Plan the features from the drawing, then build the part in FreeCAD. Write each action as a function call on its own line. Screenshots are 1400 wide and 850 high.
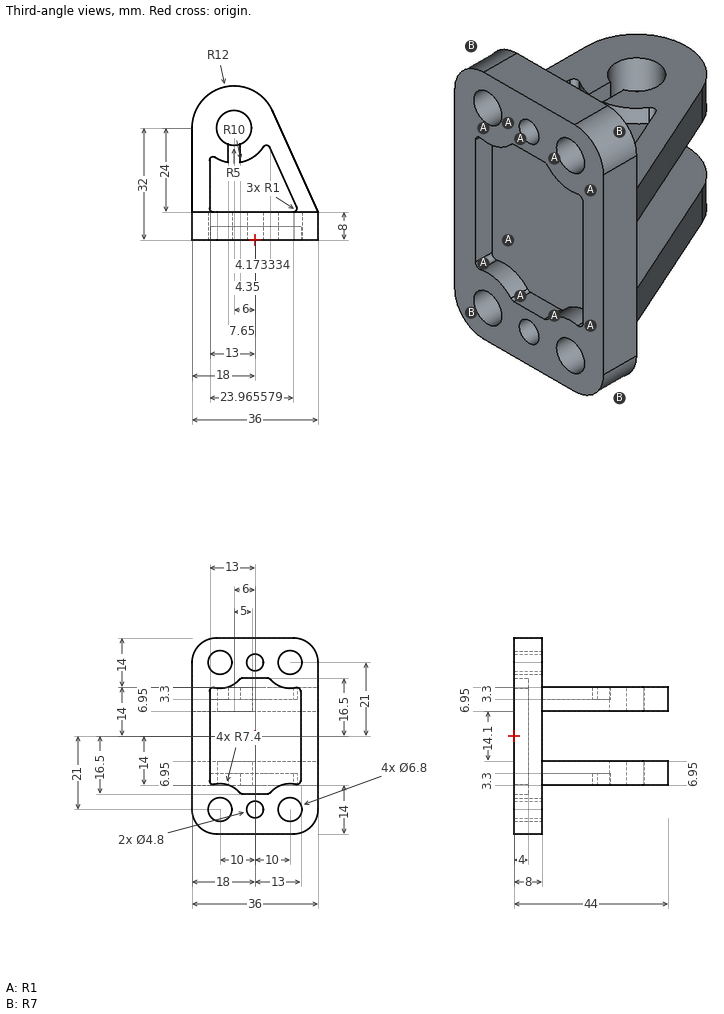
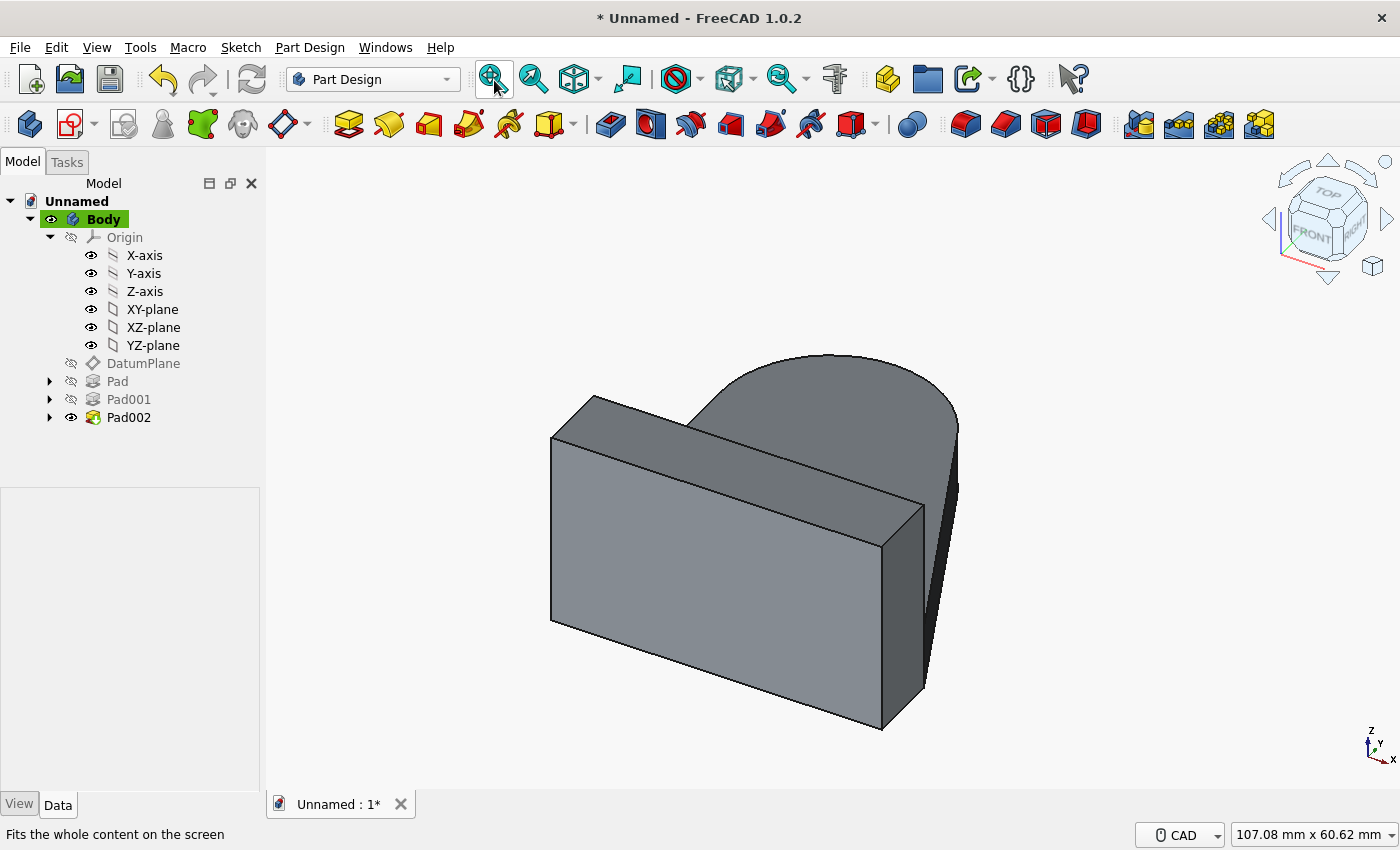
click(832, 502)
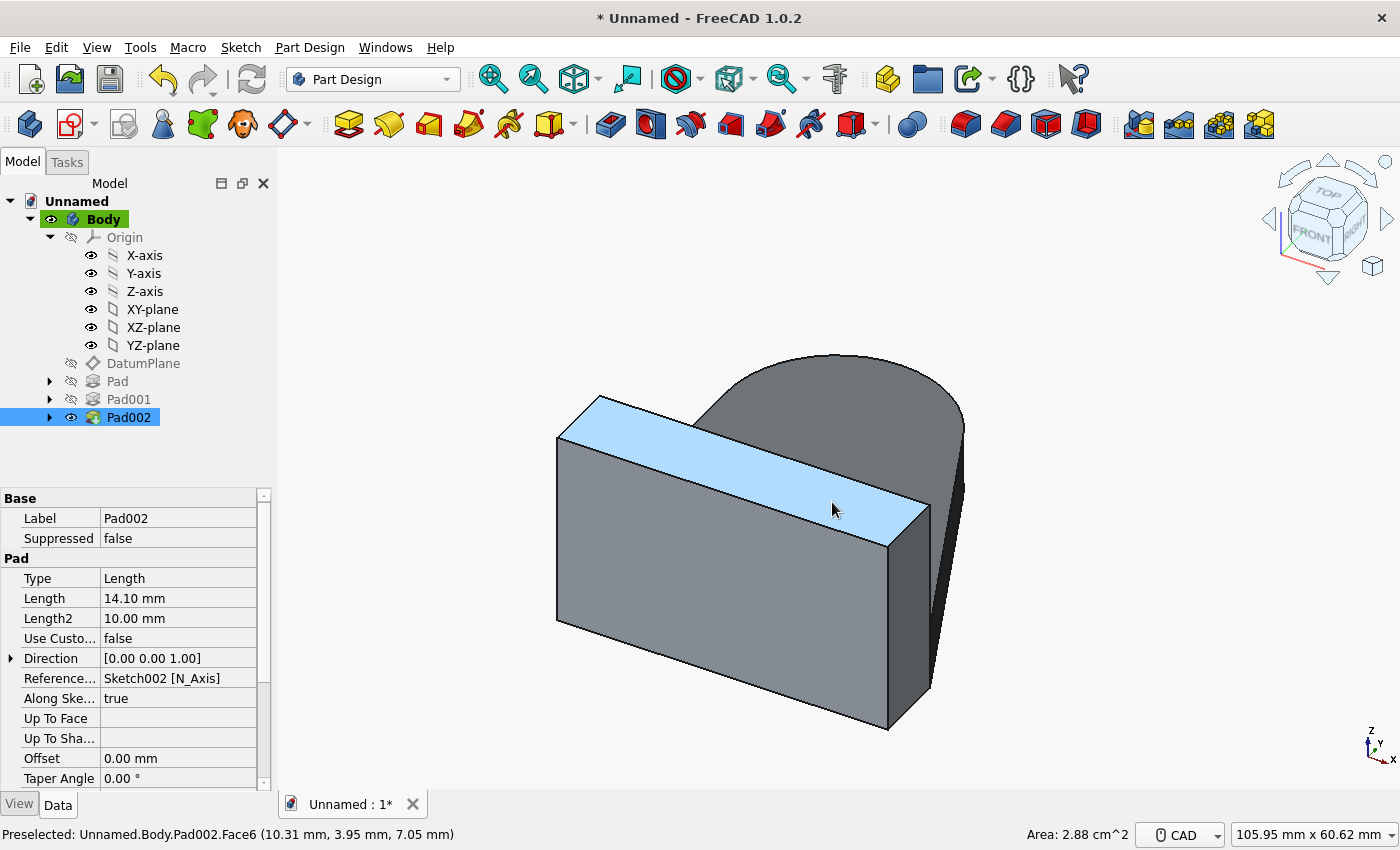
click(70, 124)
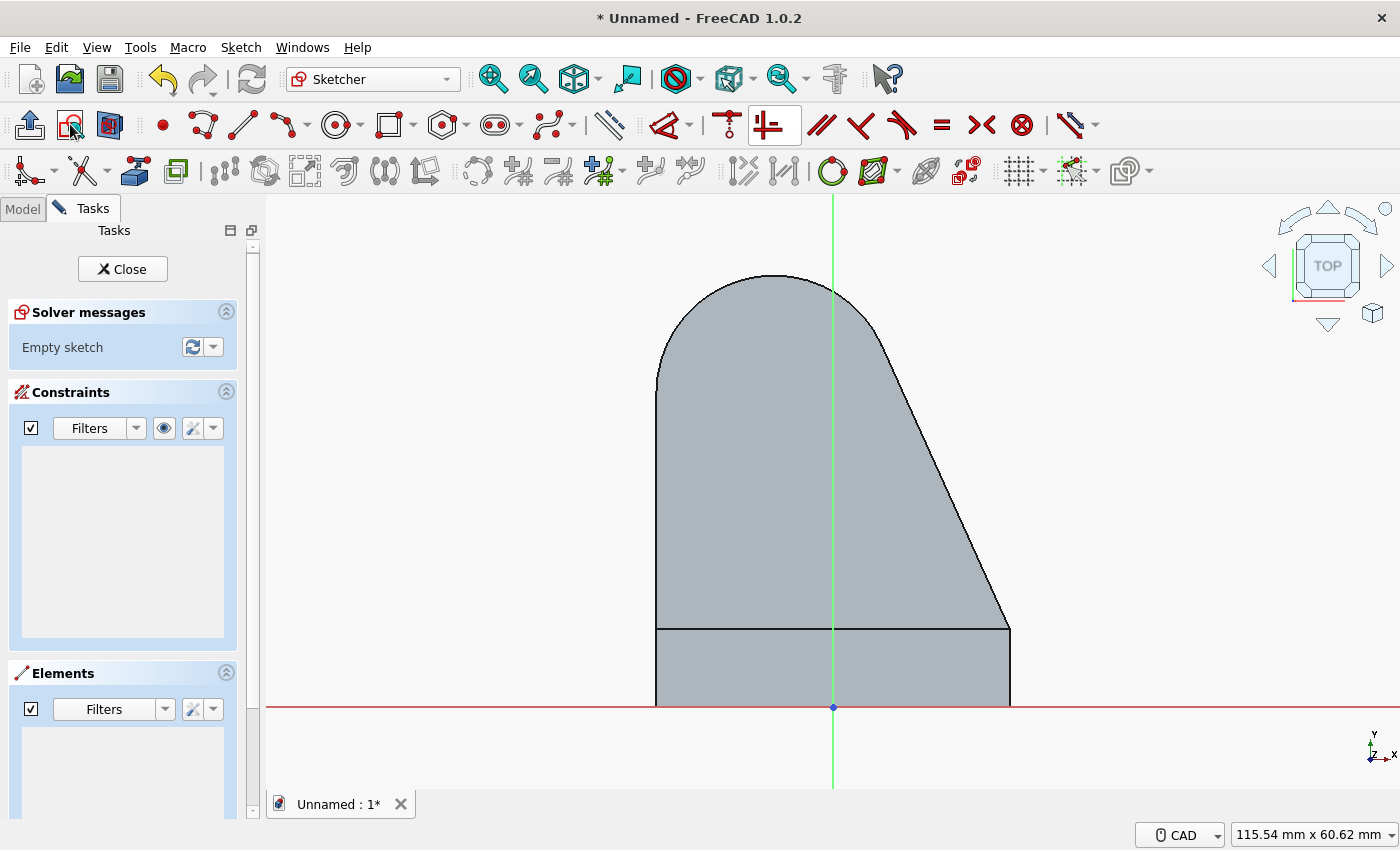
key(g)
key(m)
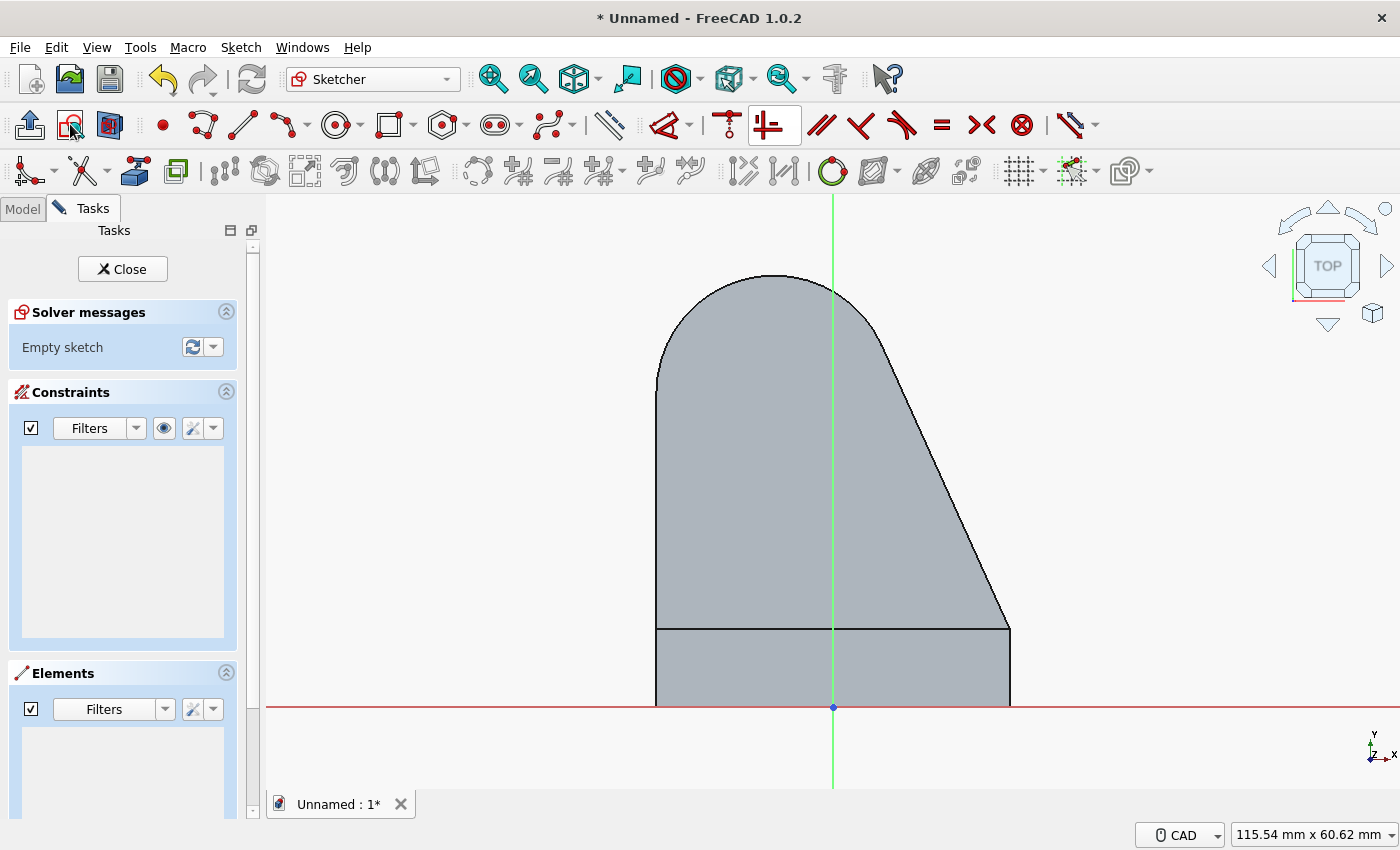
click(656, 393)
click(656, 707)
click(1010, 698)
click(1010, 629)
click(881, 345)
right_click(881, 345)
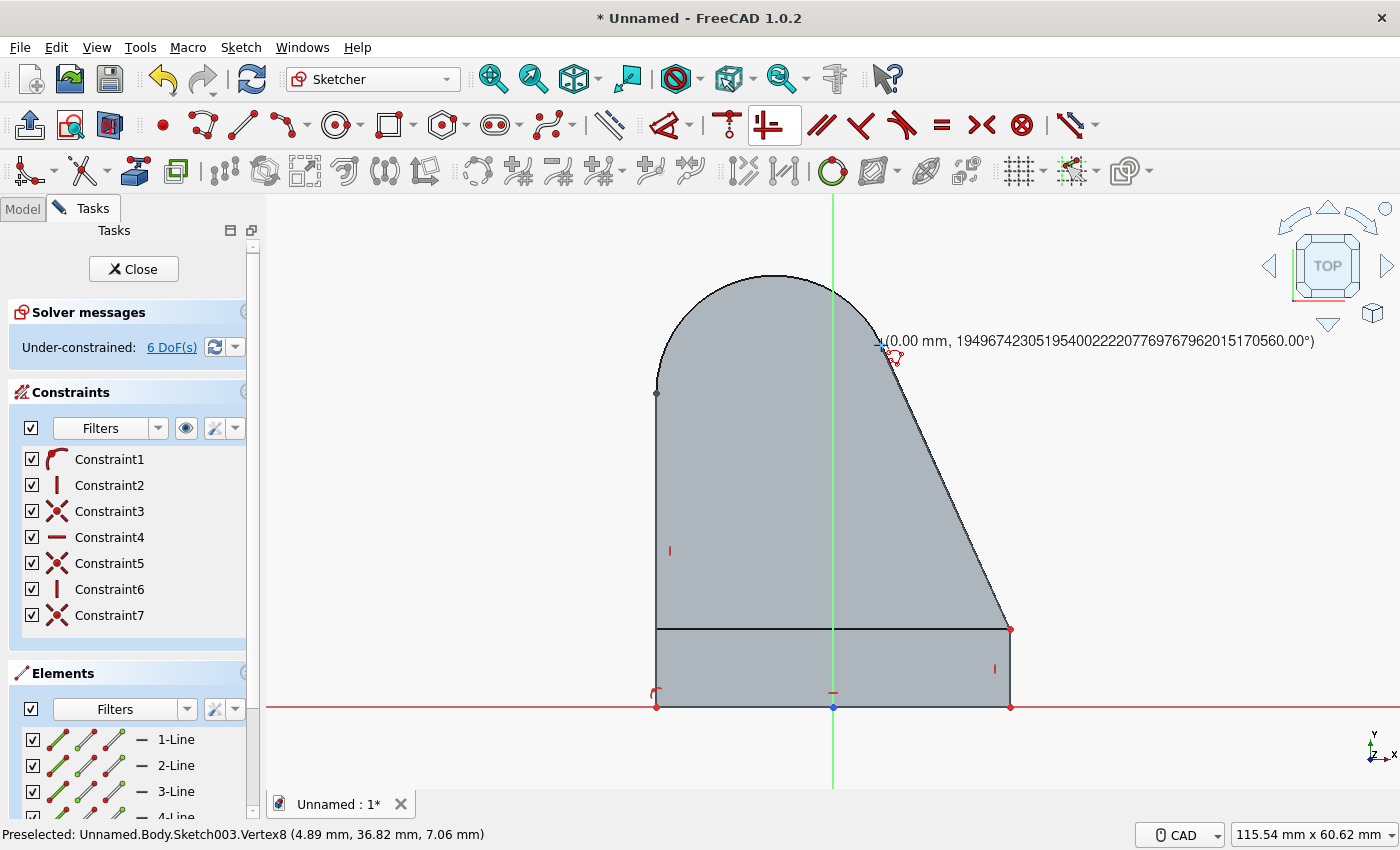
key(g)
key(3)
key(a)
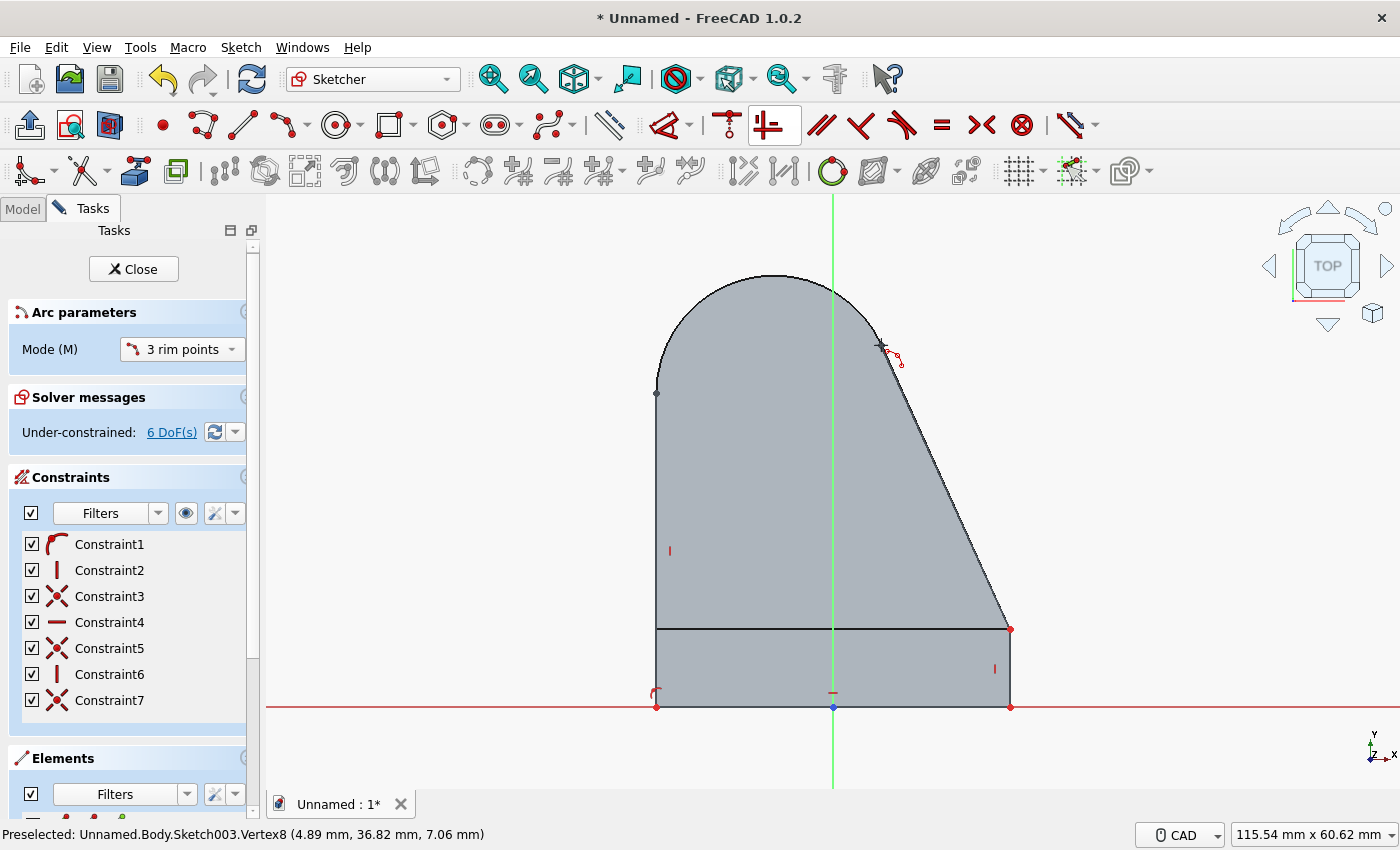
click(881, 346)
click(656, 394)
click(749, 278)
key(Escape)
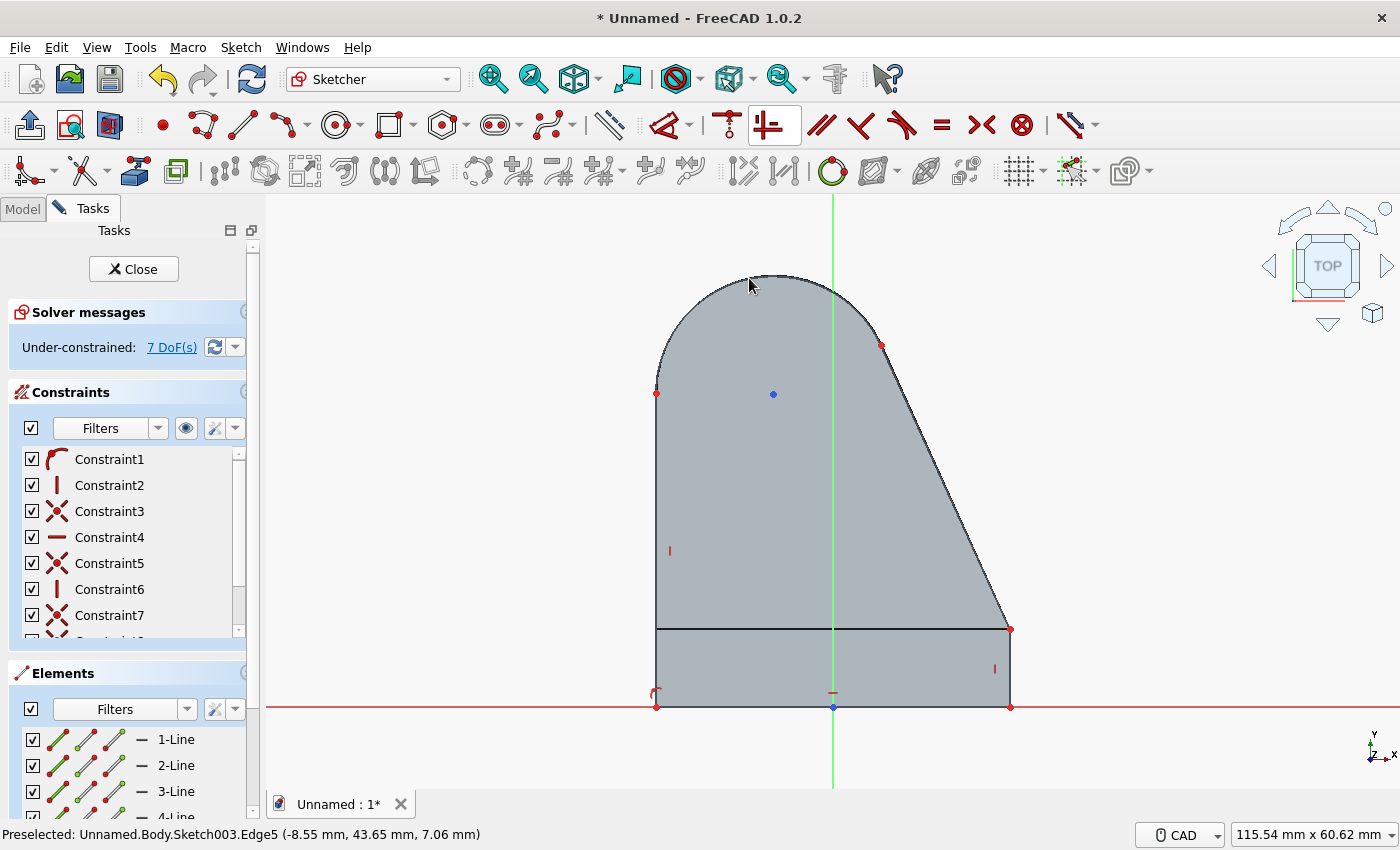
click(656, 488)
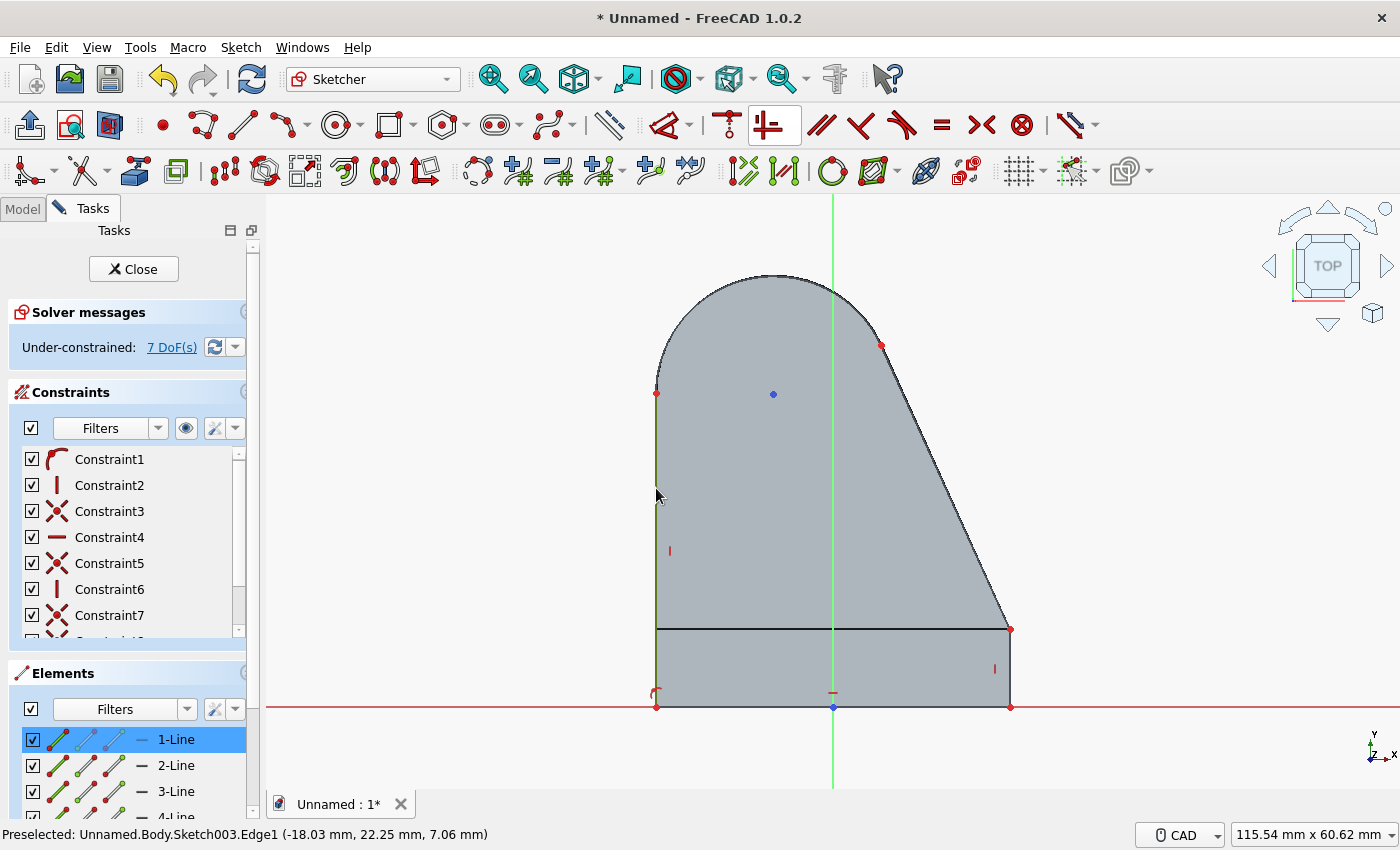
click(812, 283)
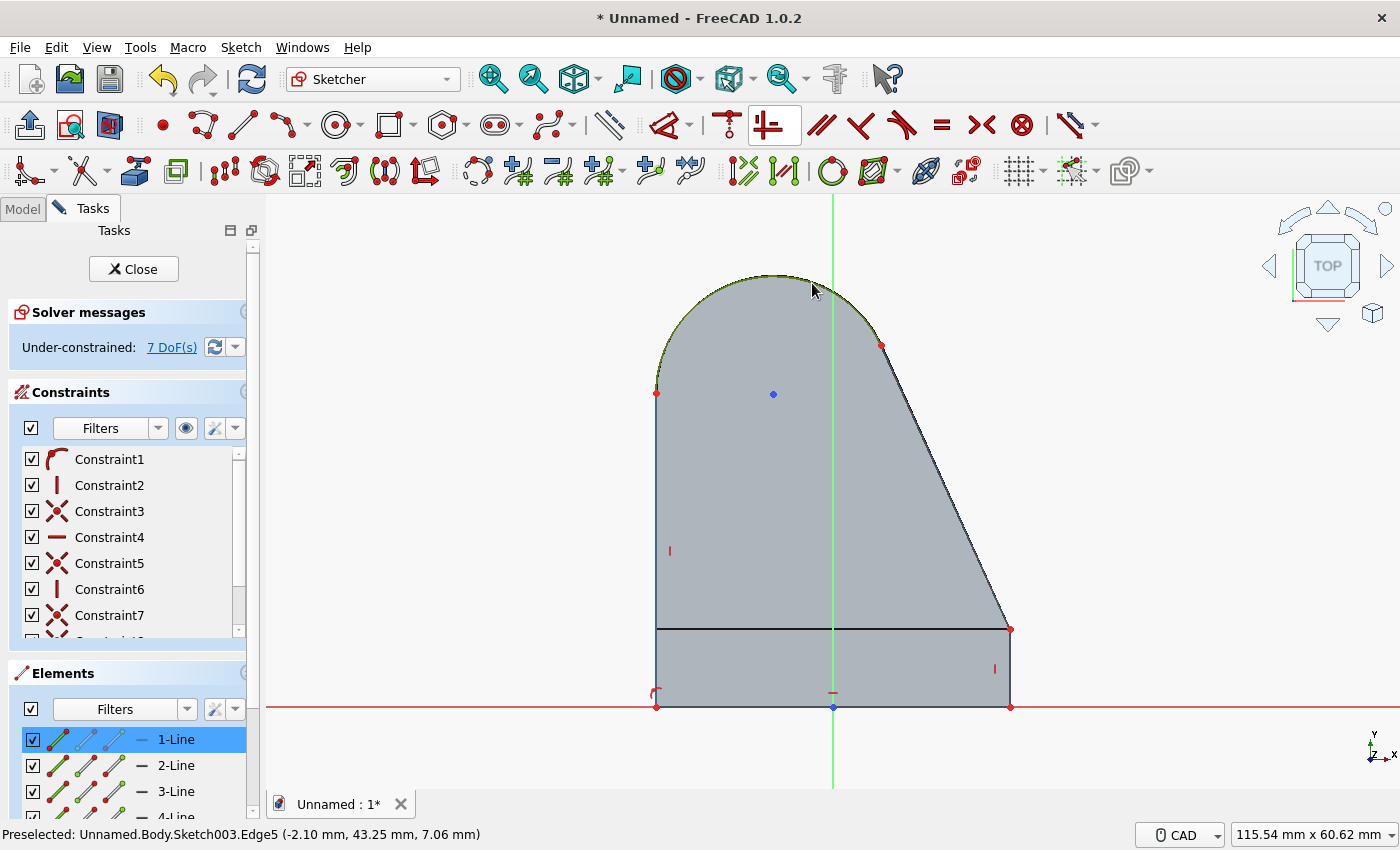
click(902, 126)